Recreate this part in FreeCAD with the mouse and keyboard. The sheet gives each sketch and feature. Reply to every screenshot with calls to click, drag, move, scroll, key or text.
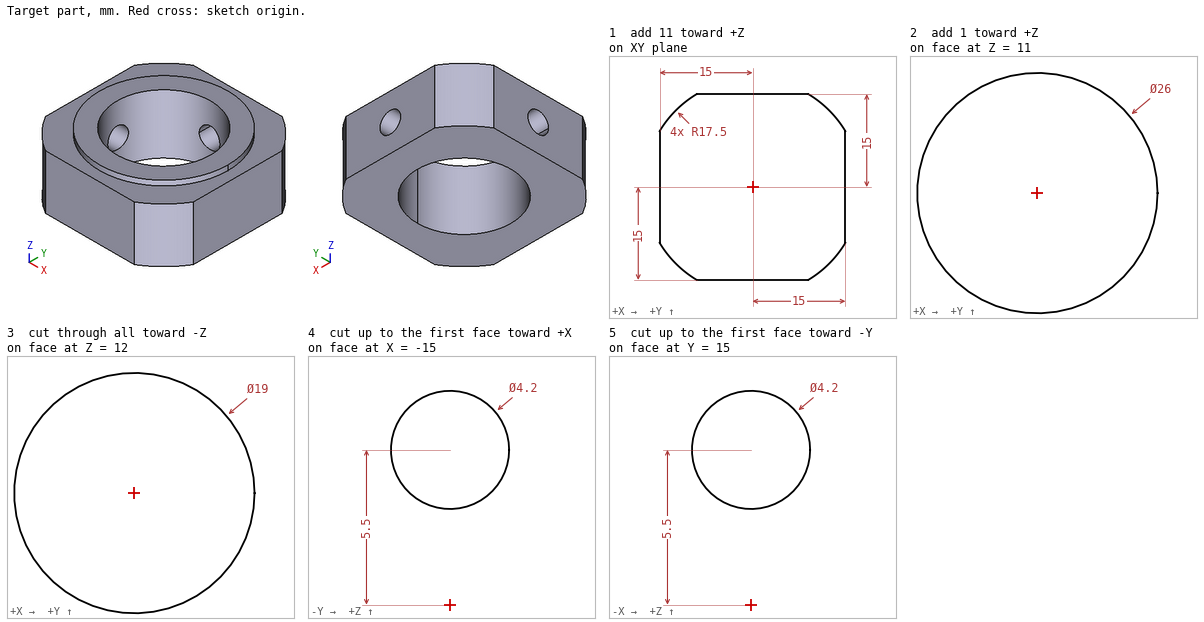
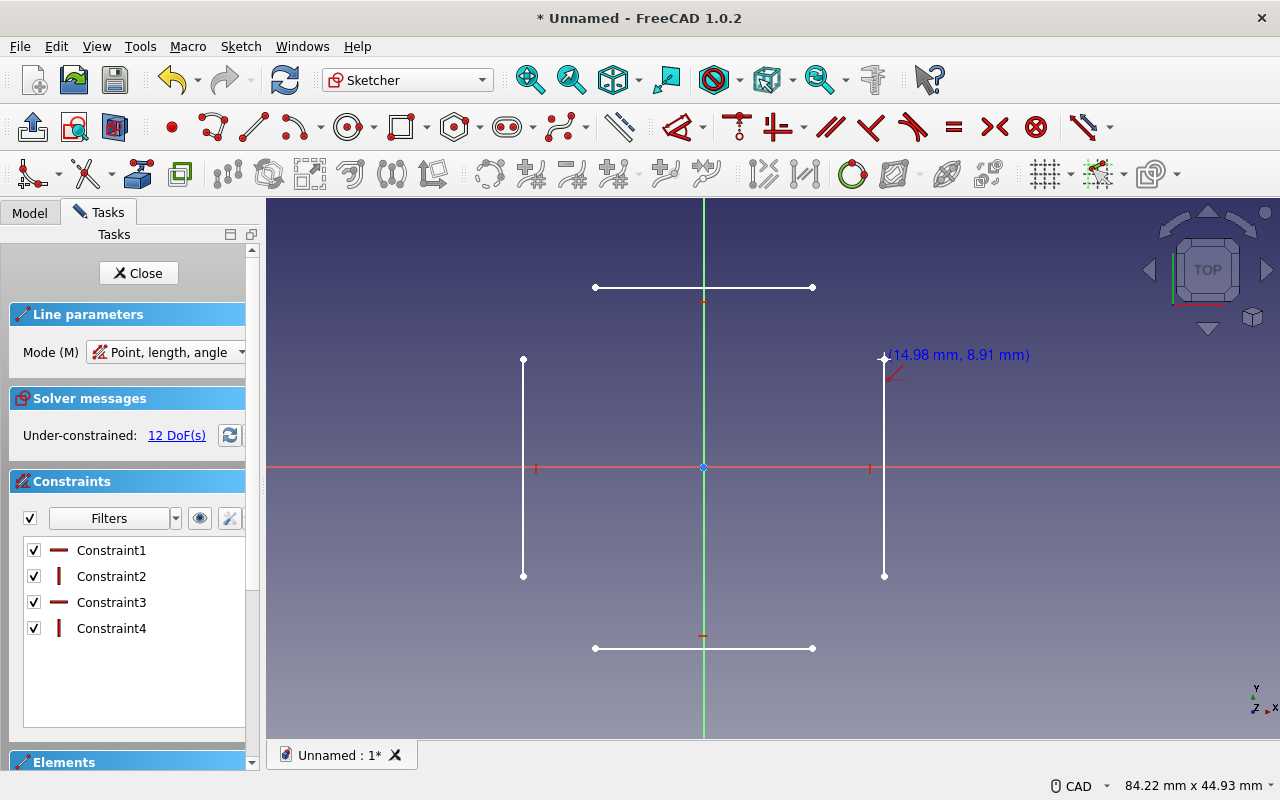
click(320, 128)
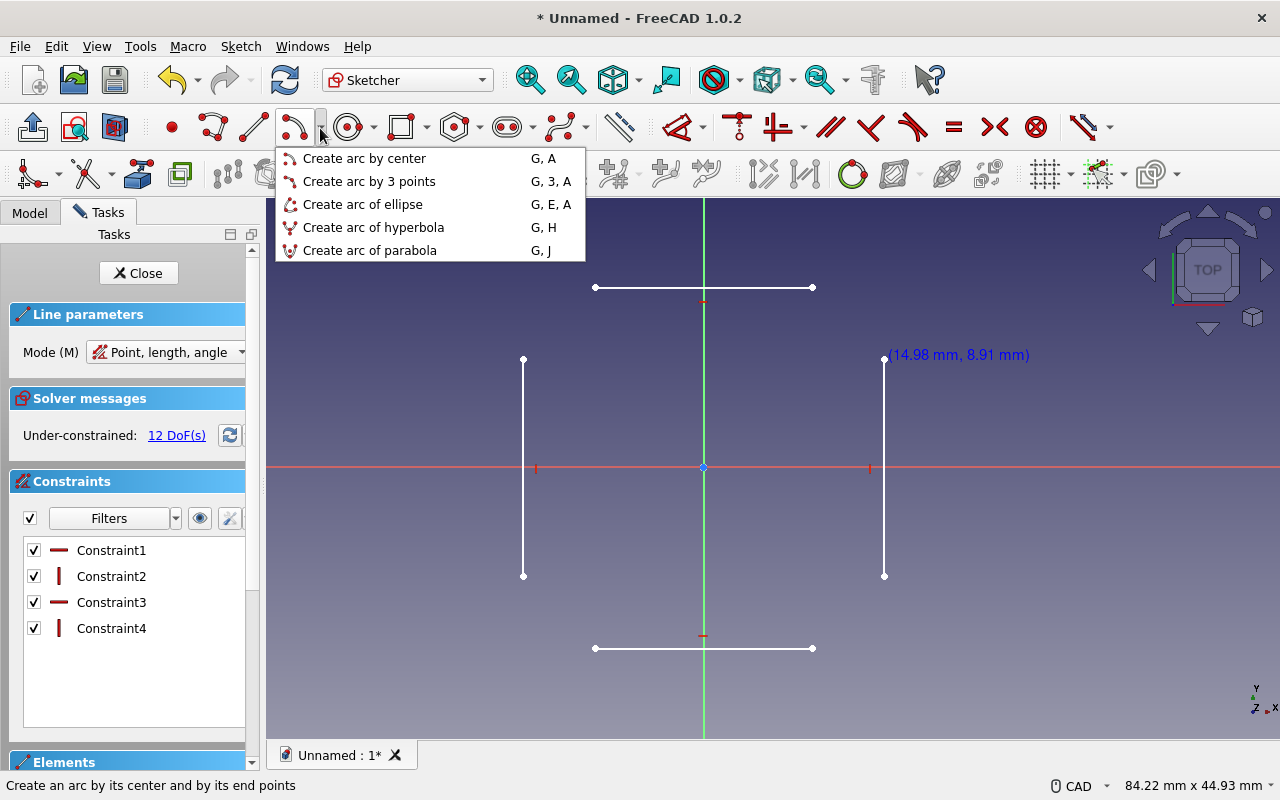
click(430, 182)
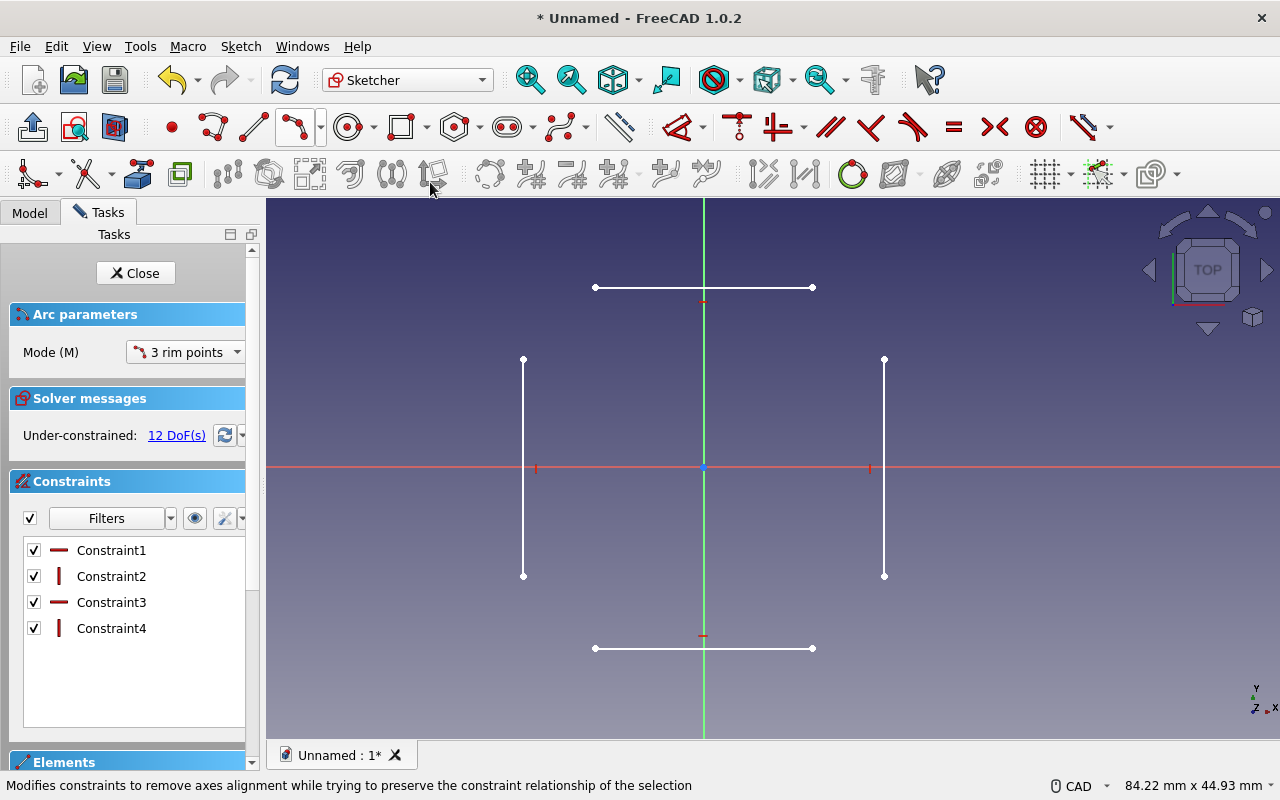
click(595, 288)
click(523, 360)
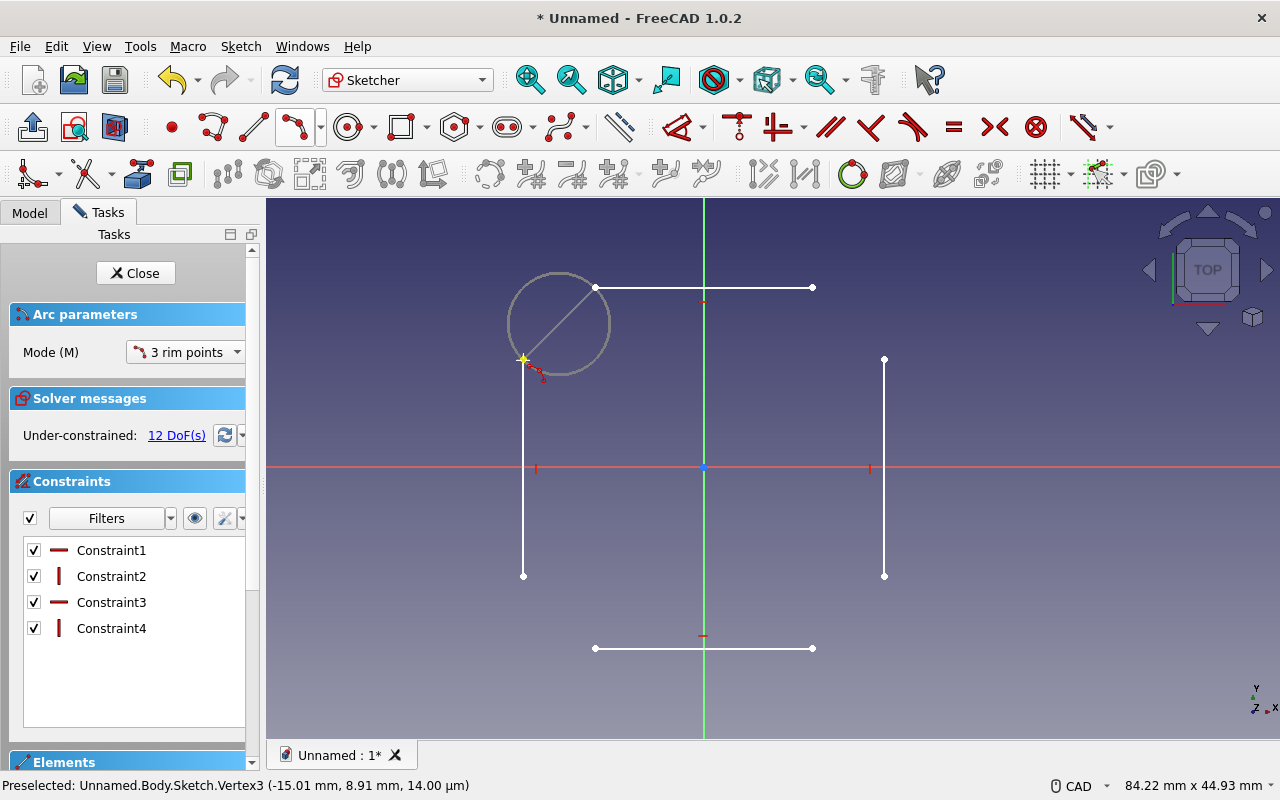
scroll(555, 318, up, 5)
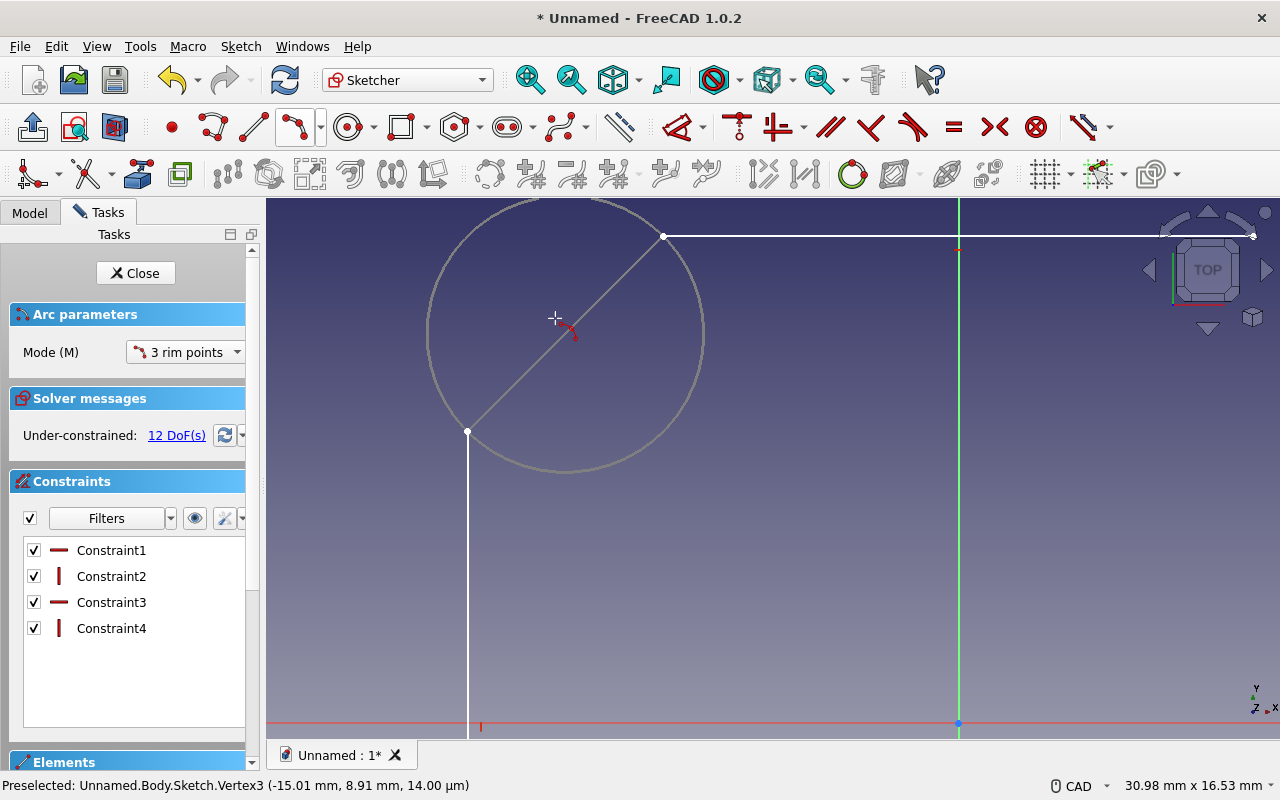
click(554, 318)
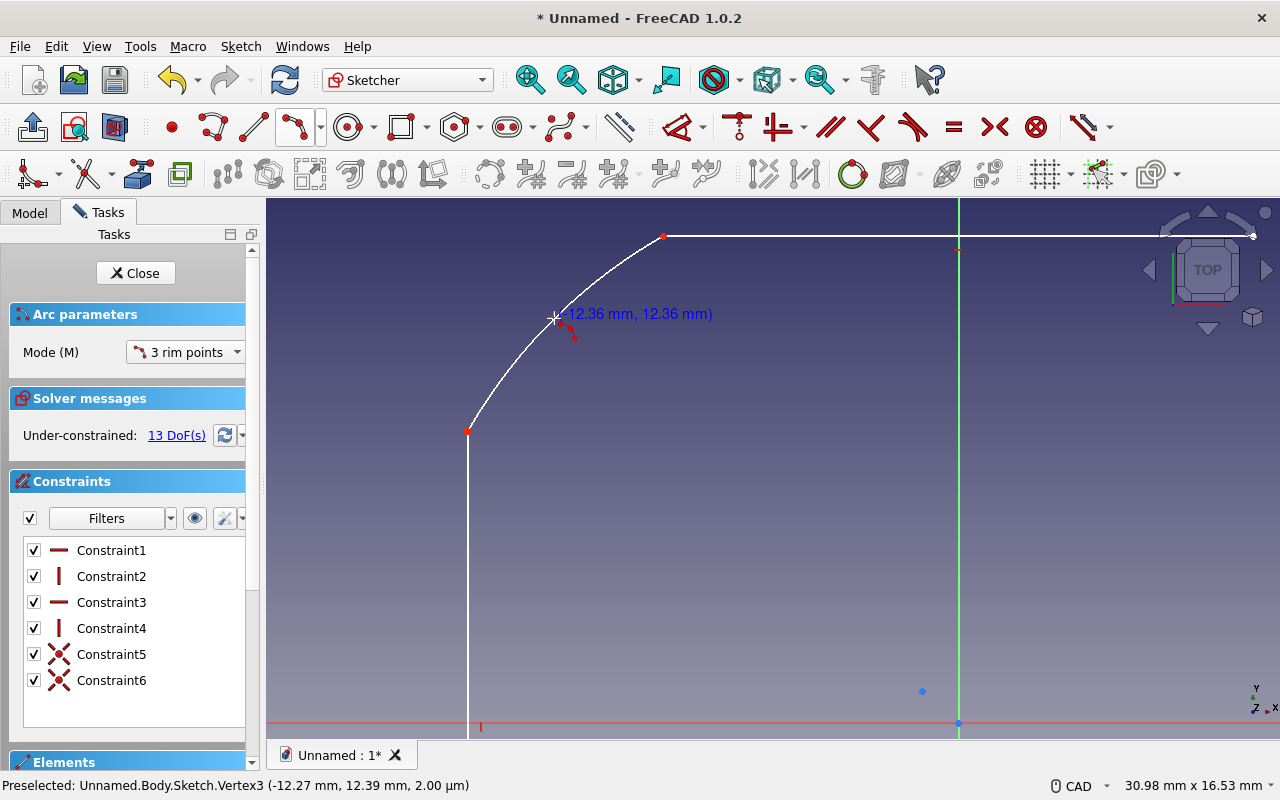
scroll(557, 320, down, 5)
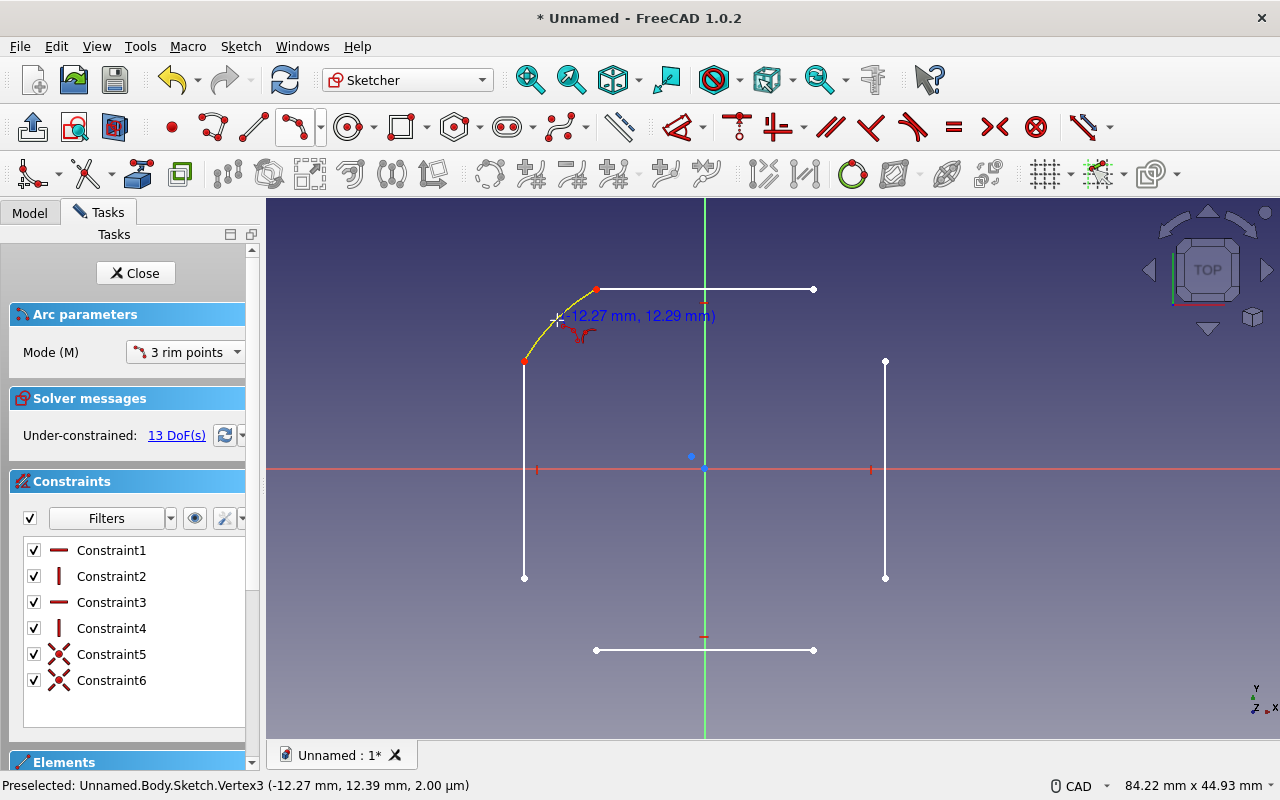
click(524, 578)
click(596, 650)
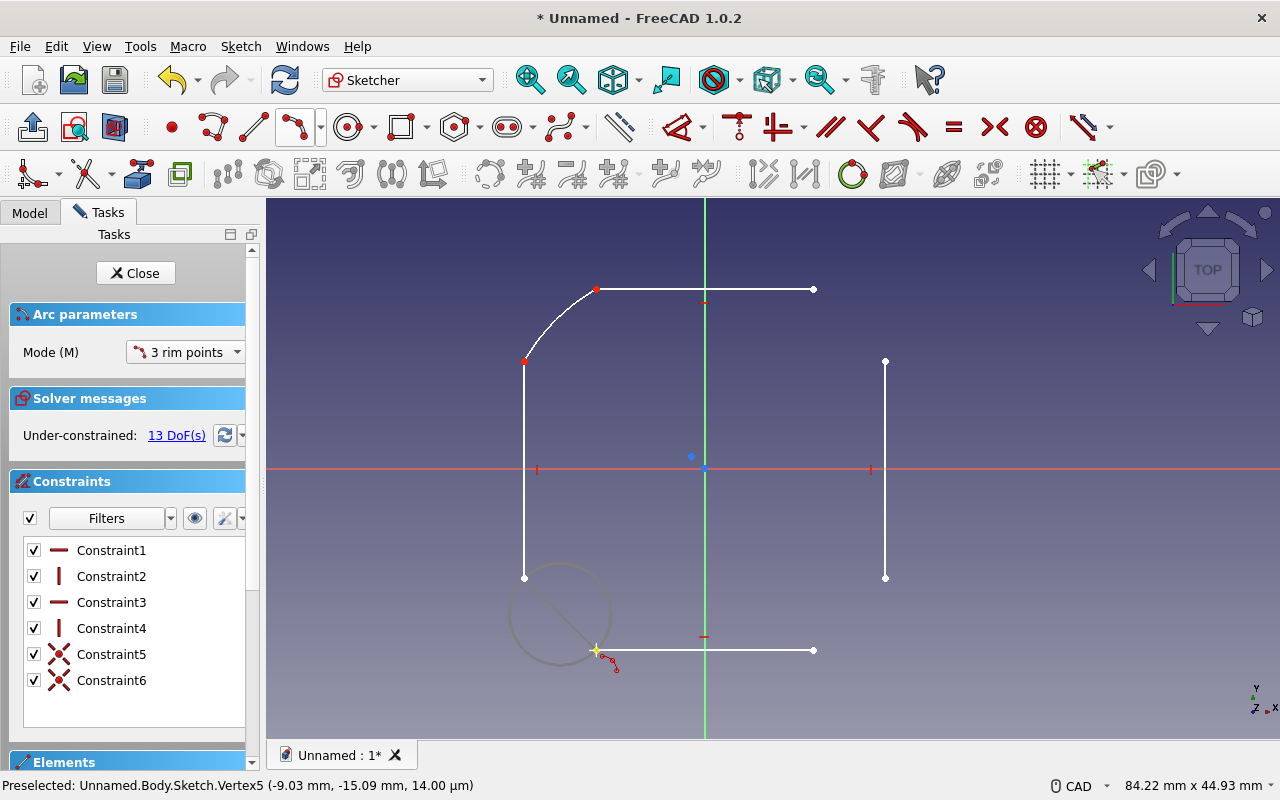
scroll(556, 618, up, 5)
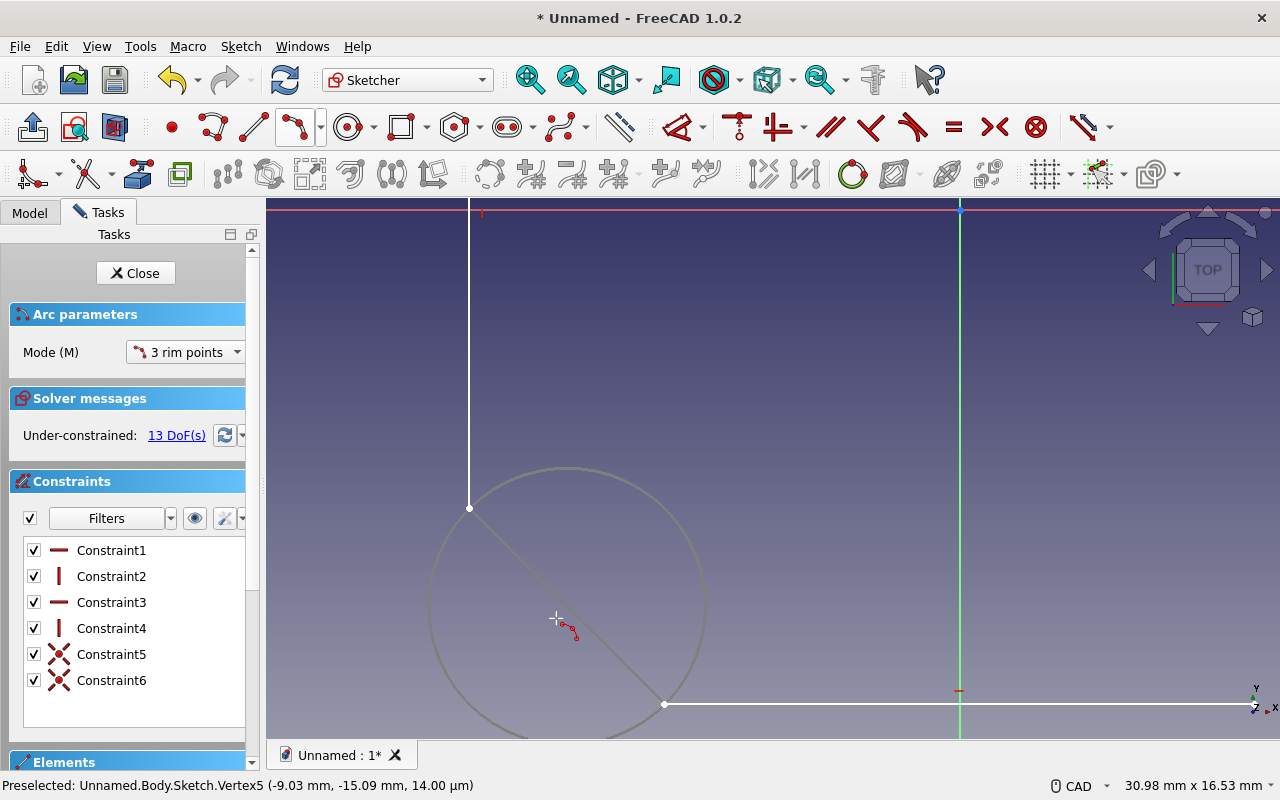
click(555, 615)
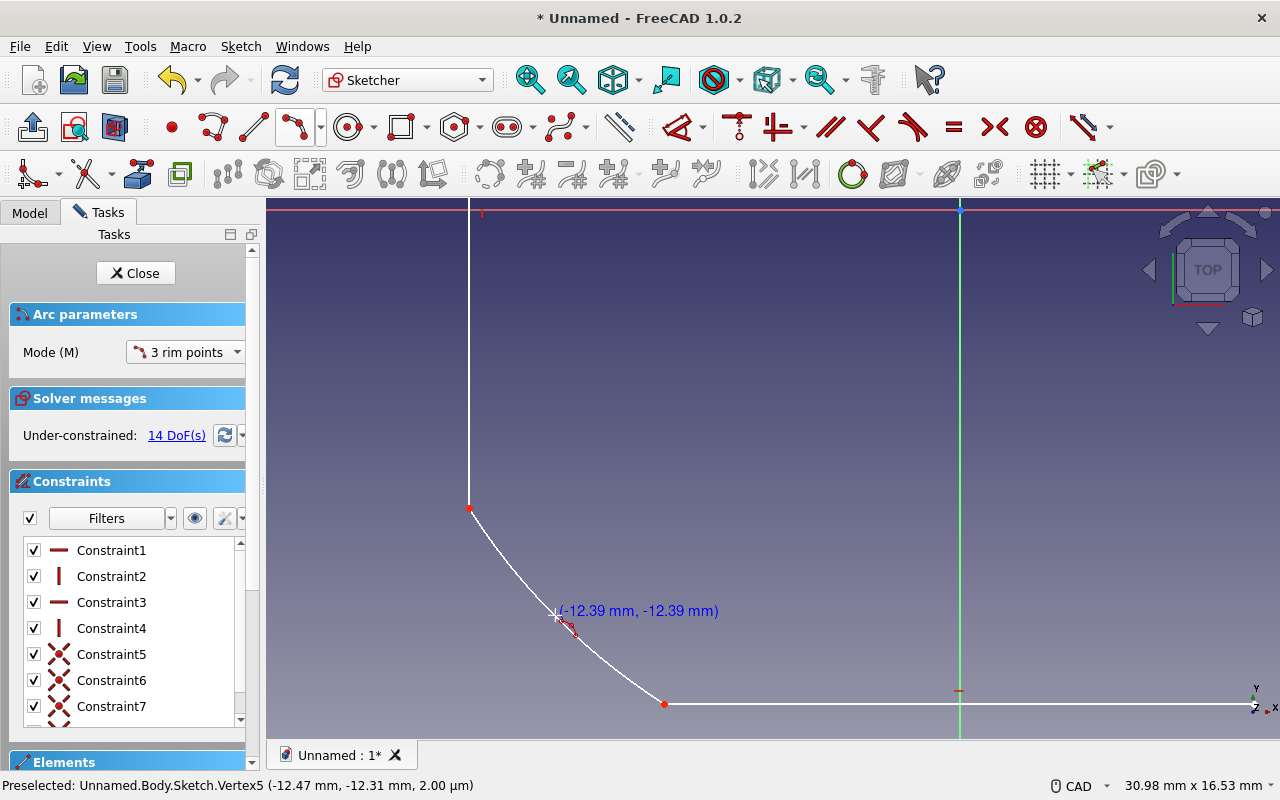
scroll(556, 619, down, 5)